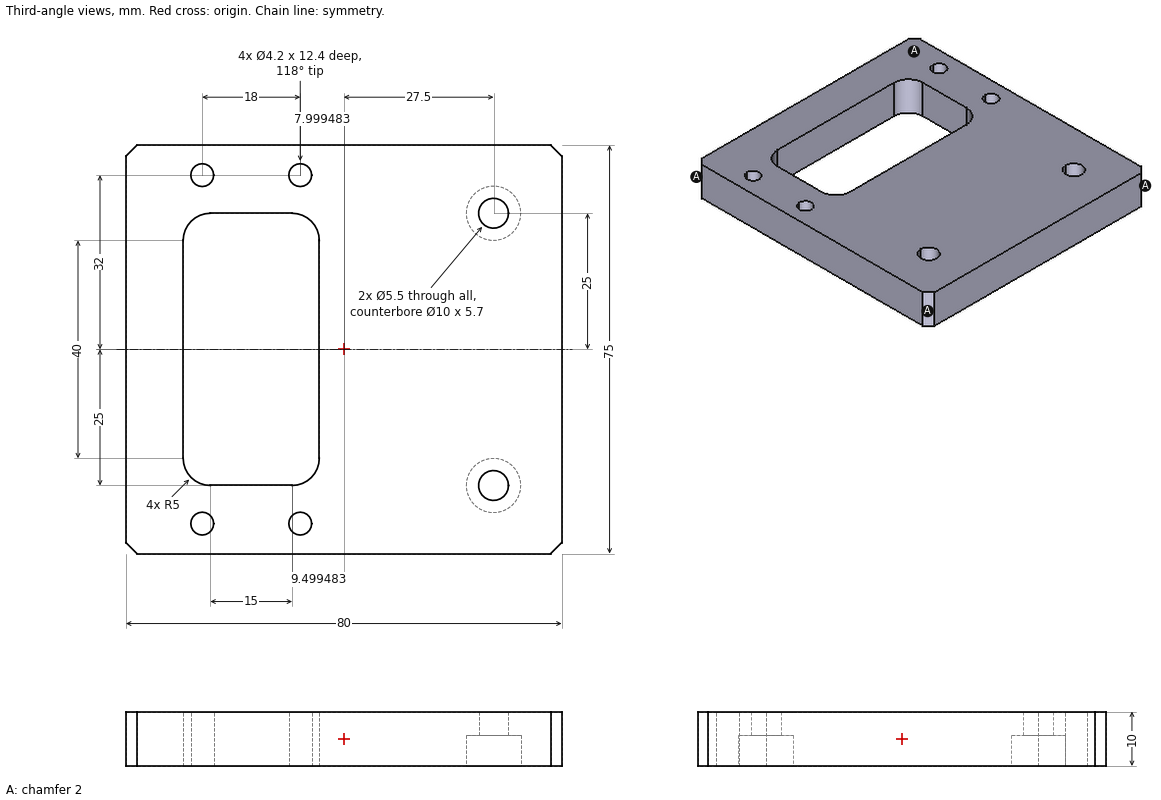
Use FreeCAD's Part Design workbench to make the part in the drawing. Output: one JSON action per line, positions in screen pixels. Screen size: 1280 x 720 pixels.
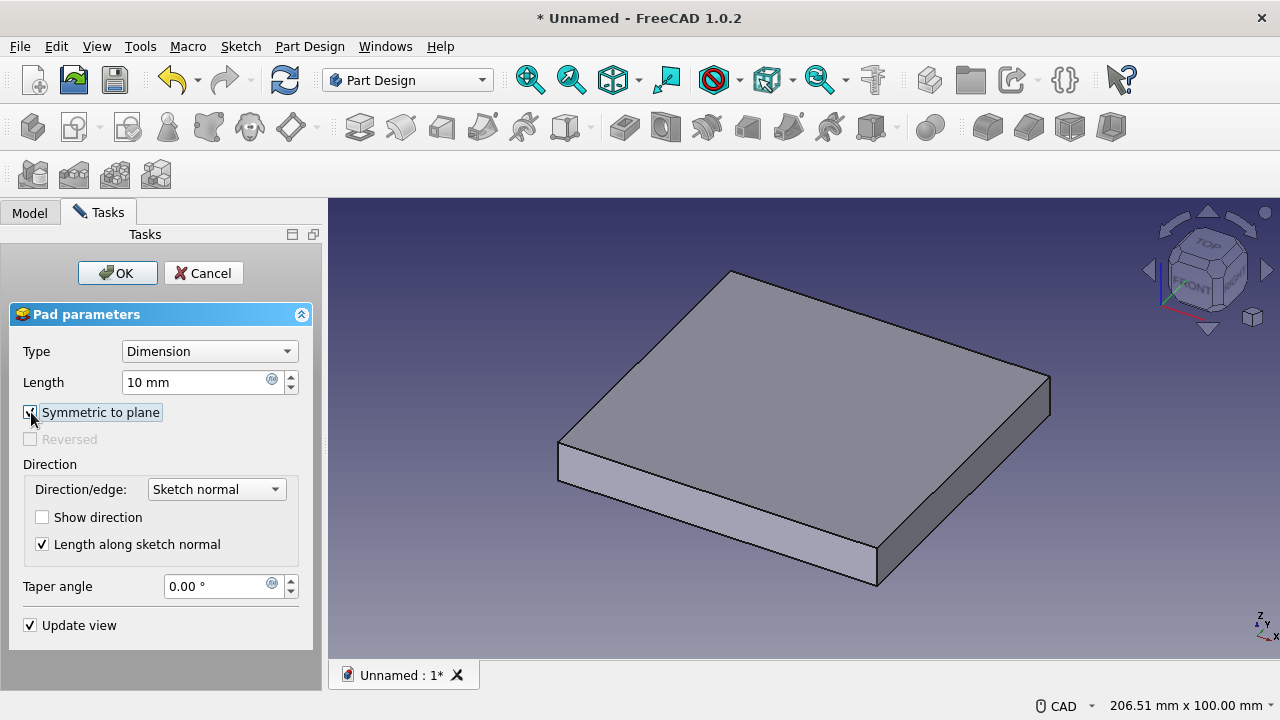
{"action": "left_click", "coordinate": [118, 273]}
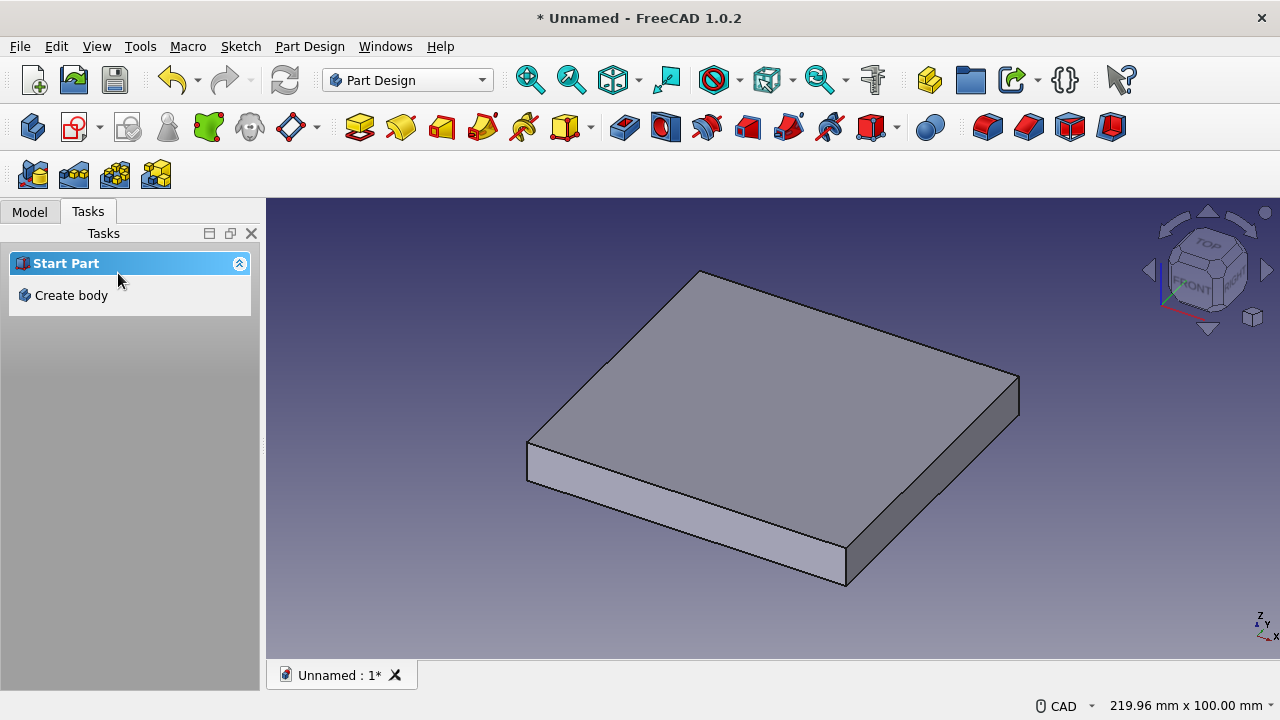
{"action": "left_click", "coordinate": [846, 566]}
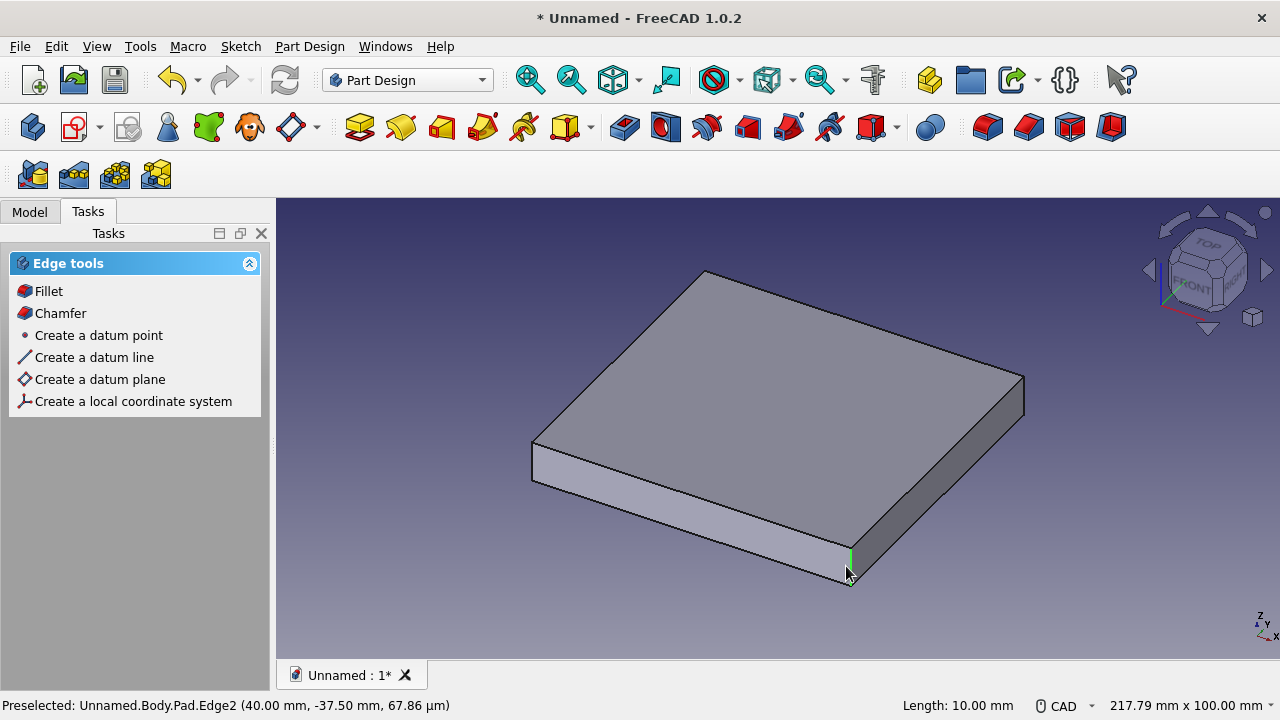
{"action": "key", "text": "0"}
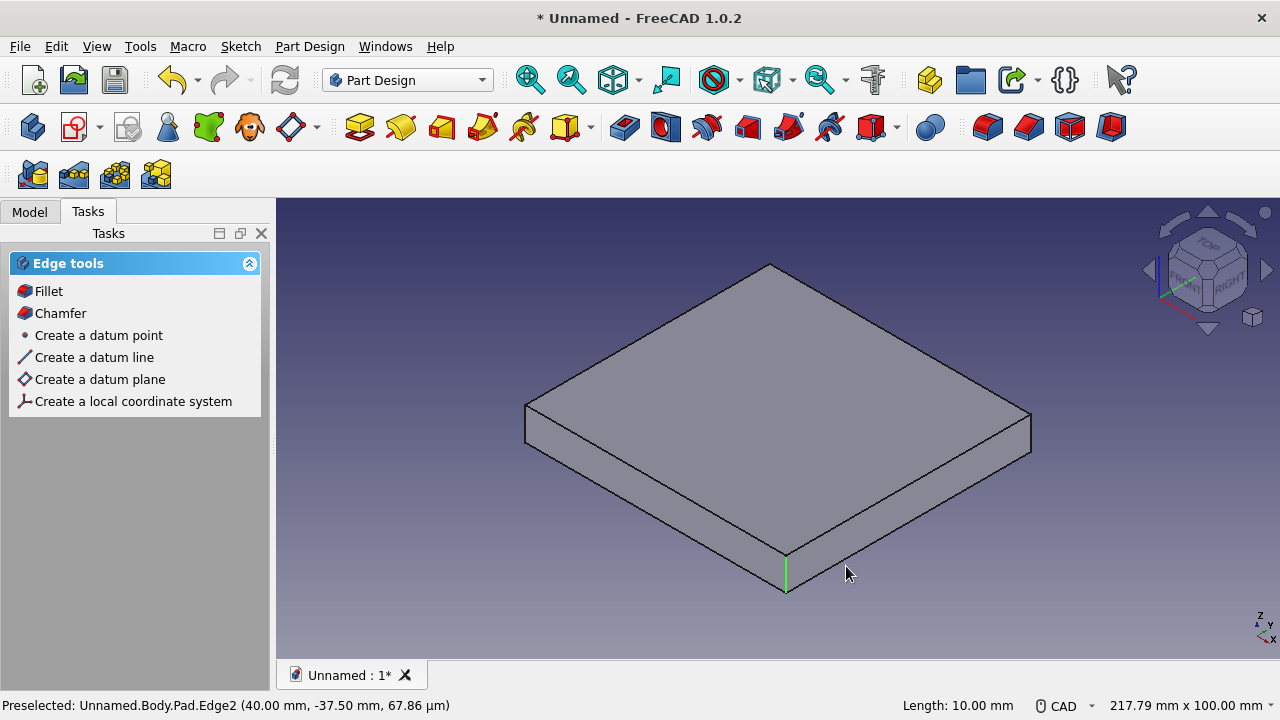
{"action": "key", "text": "2"}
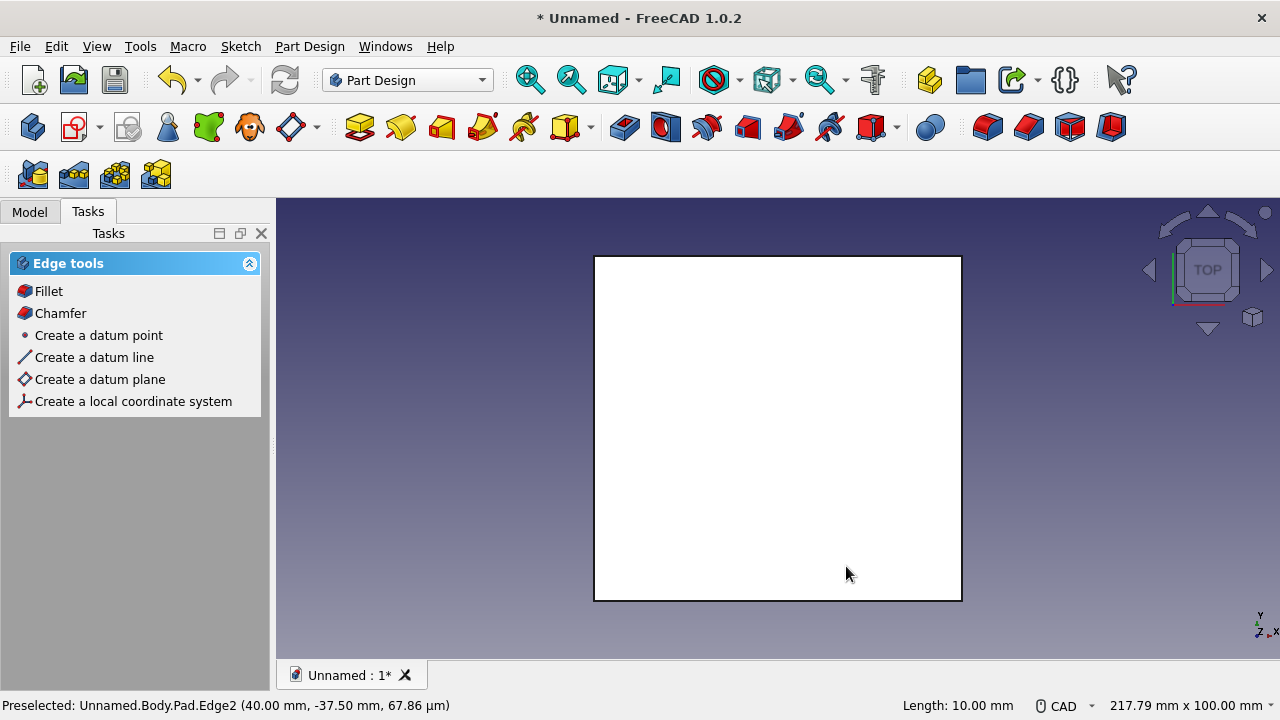
{"action": "key", "text": "1"}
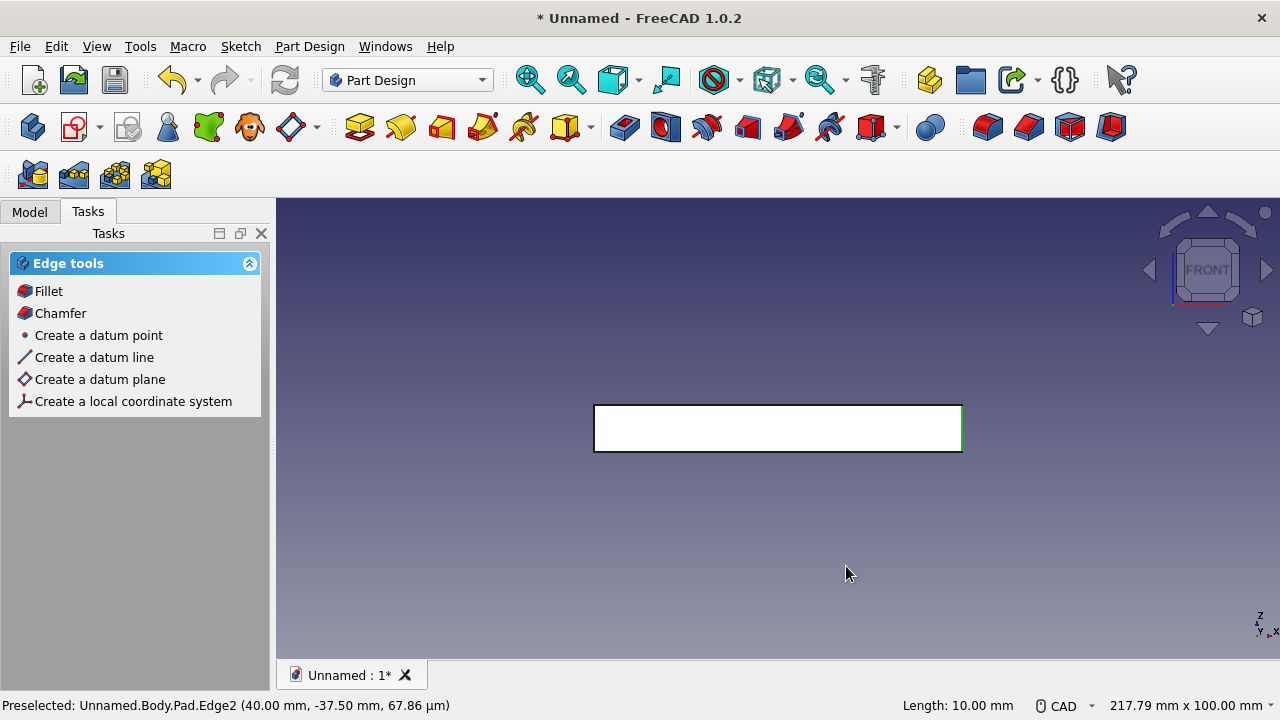
{"action": "key", "text": "v f"}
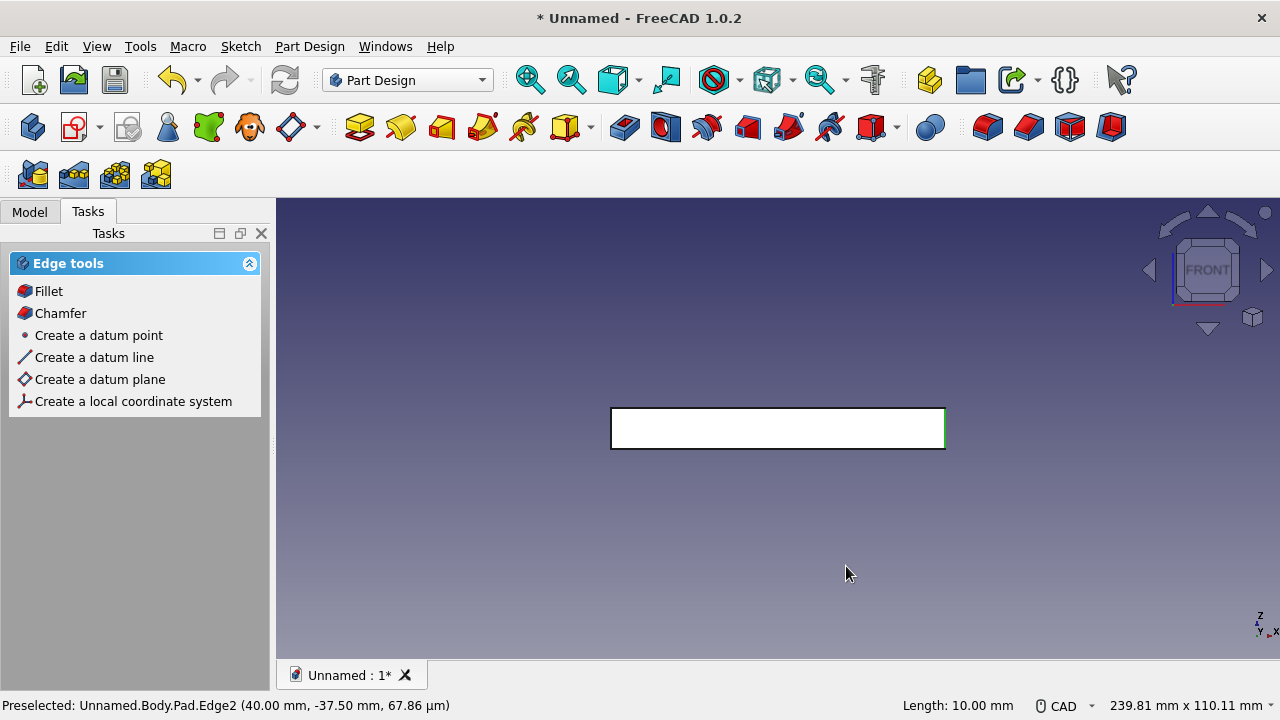
{"action": "left_click", "coordinate": [611, 428], "text": "ctrl"}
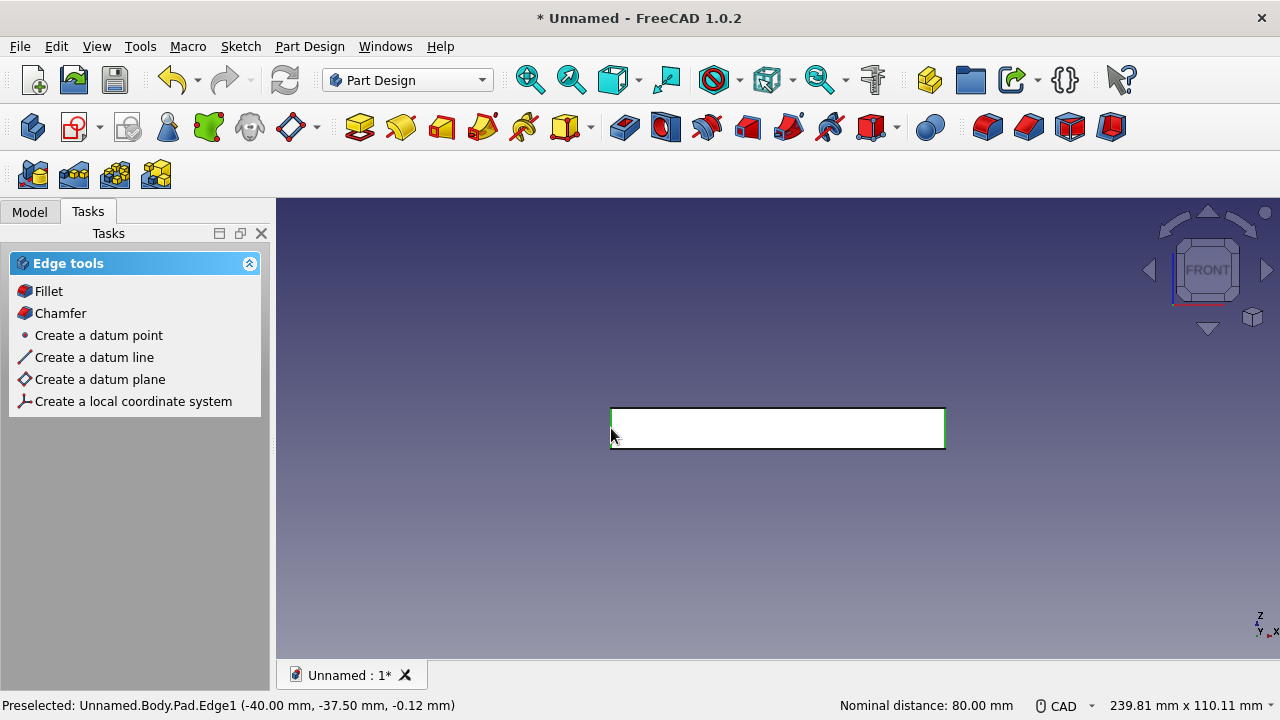
{"action": "key", "text": "3"}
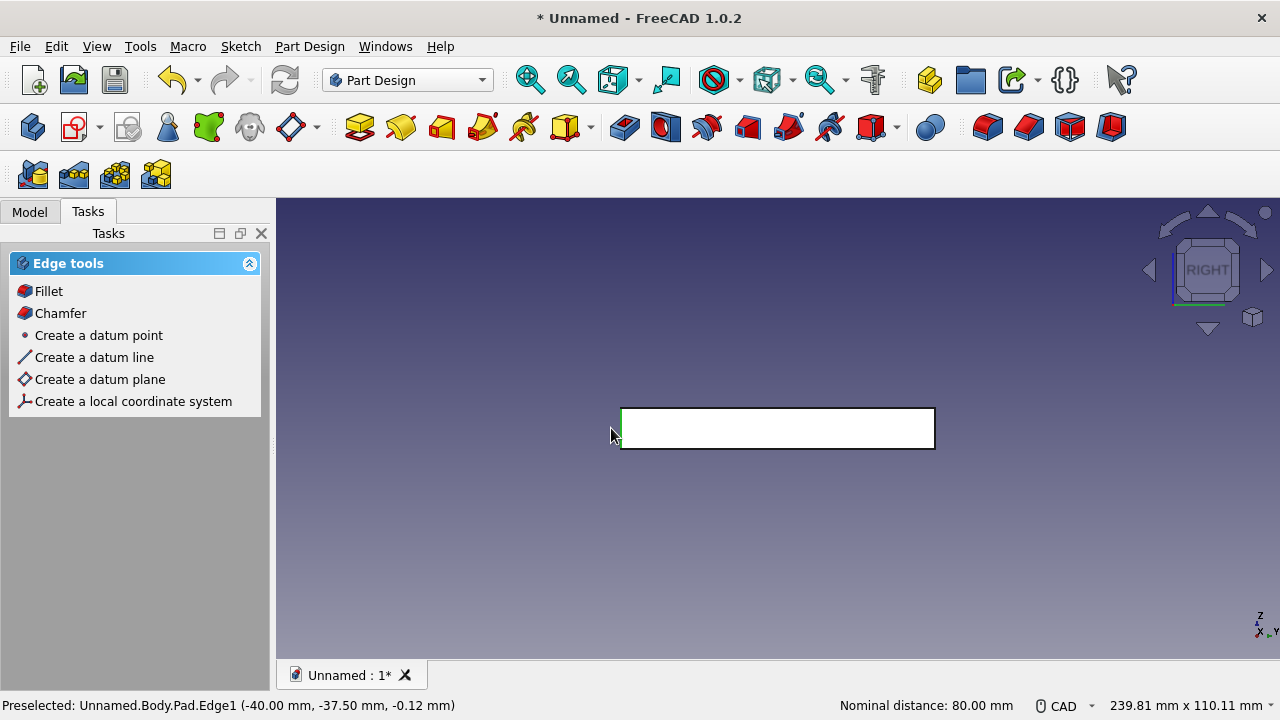
{"action": "key", "text": "v f"}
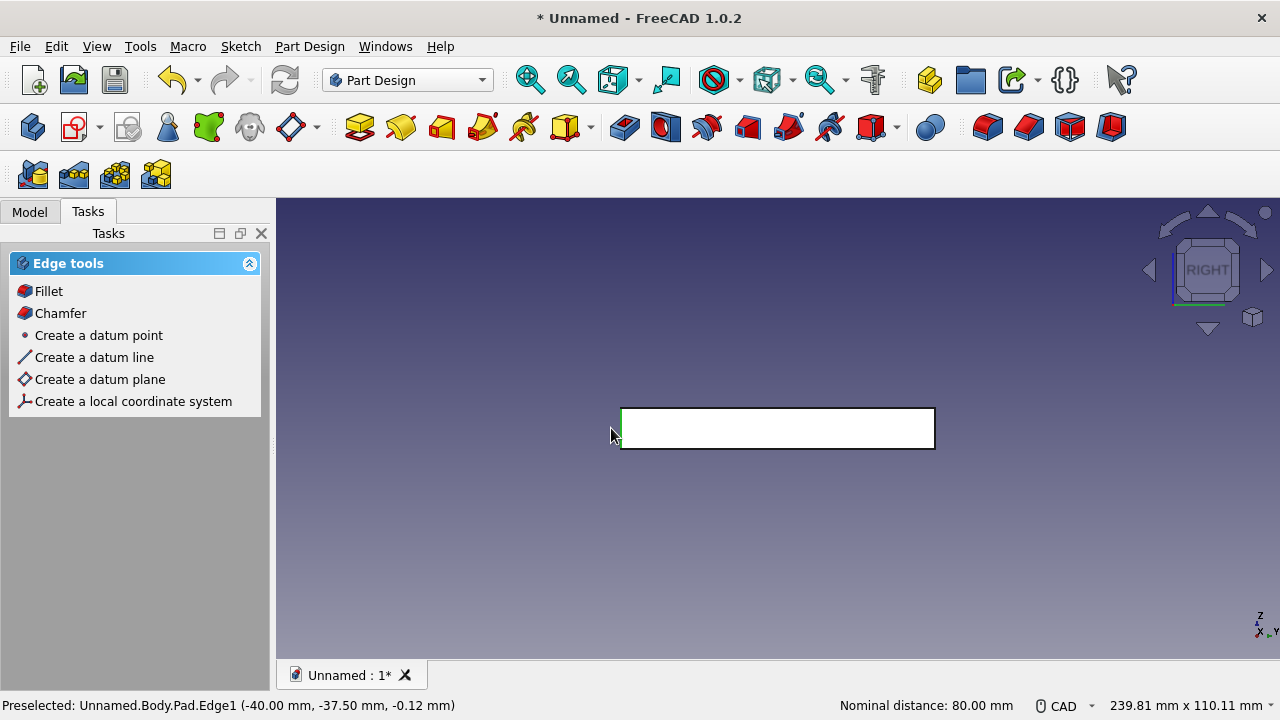
{"action": "left_click", "coordinate": [935, 427], "text": "ctrl"}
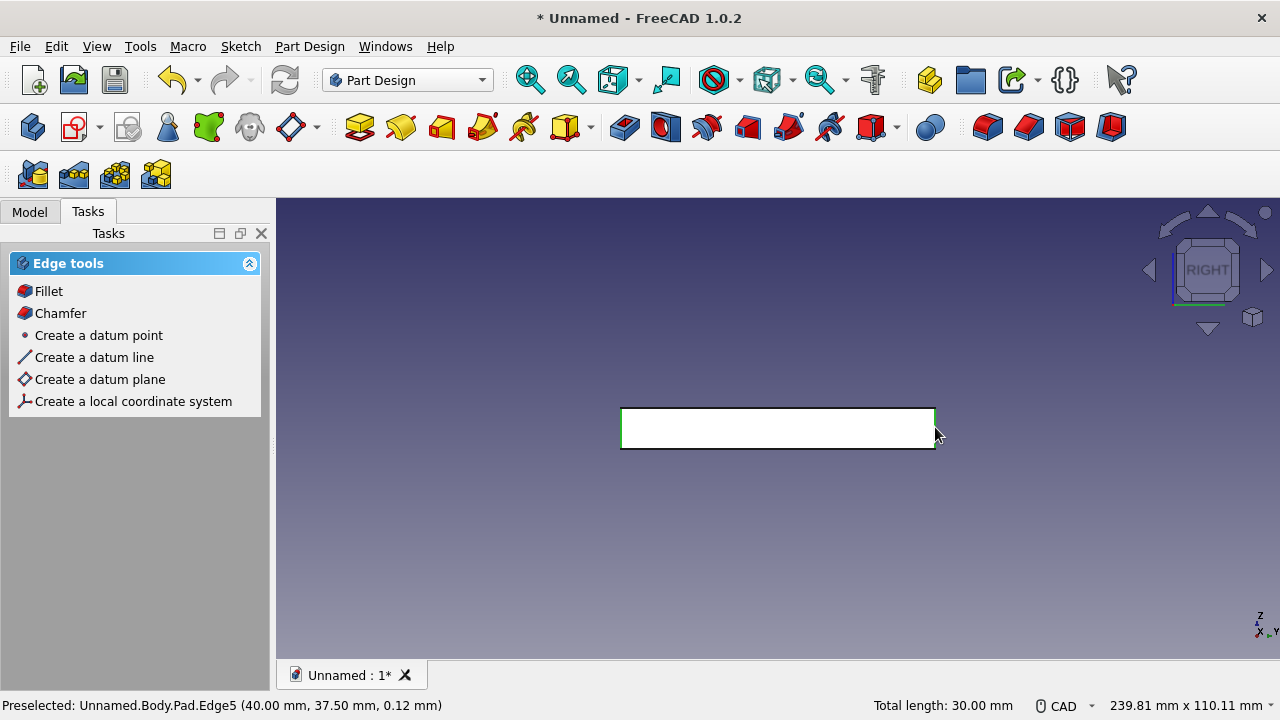
{"action": "key", "text": "5"}